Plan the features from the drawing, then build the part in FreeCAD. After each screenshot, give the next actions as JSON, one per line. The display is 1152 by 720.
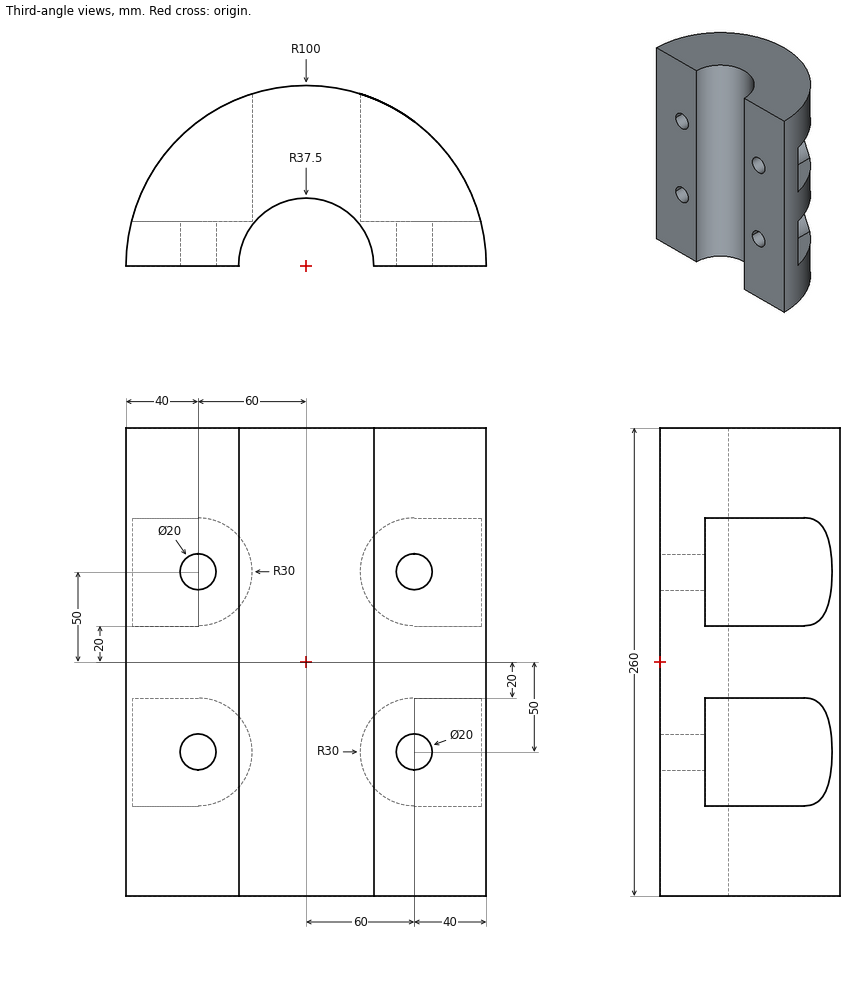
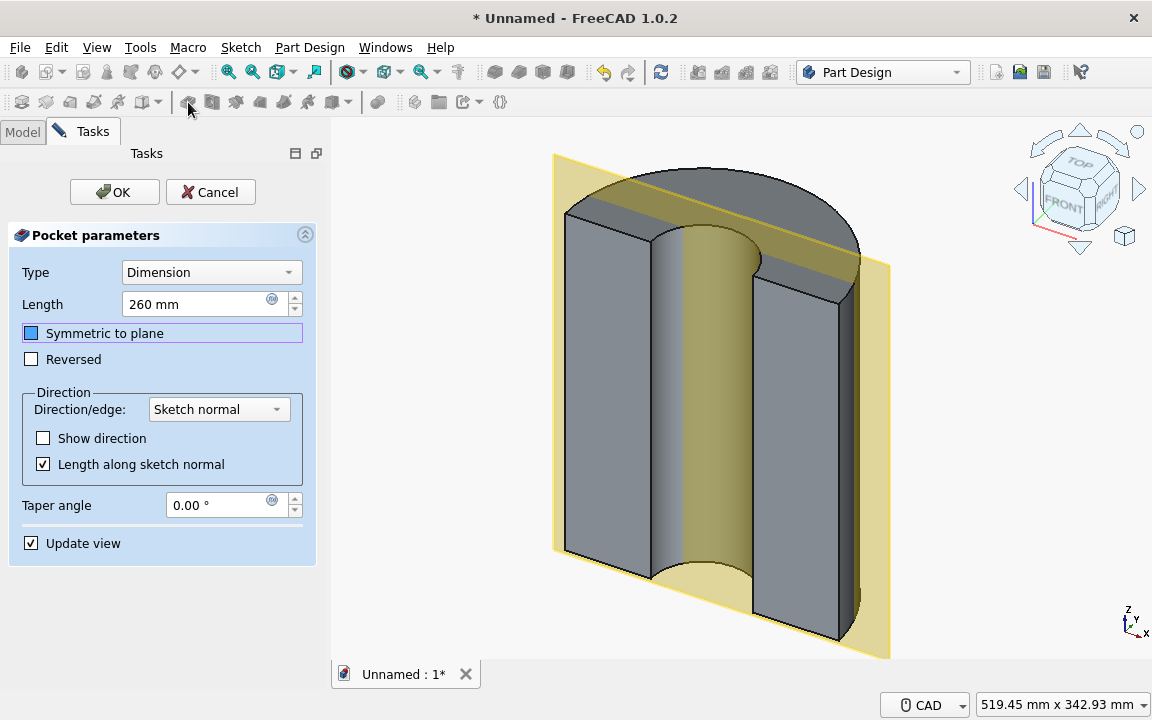
{"action": "left_click", "coordinate": [115, 192]}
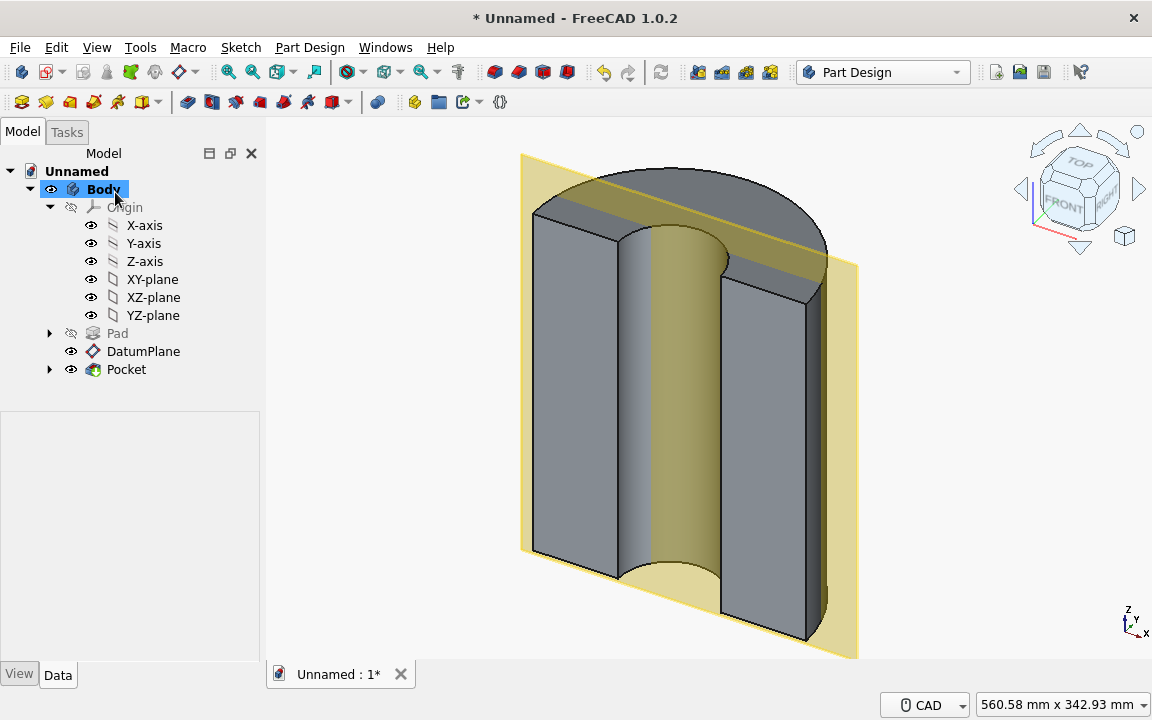
{"action": "left_click", "coordinate": [116, 351]}
{"action": "key", "text": "space"}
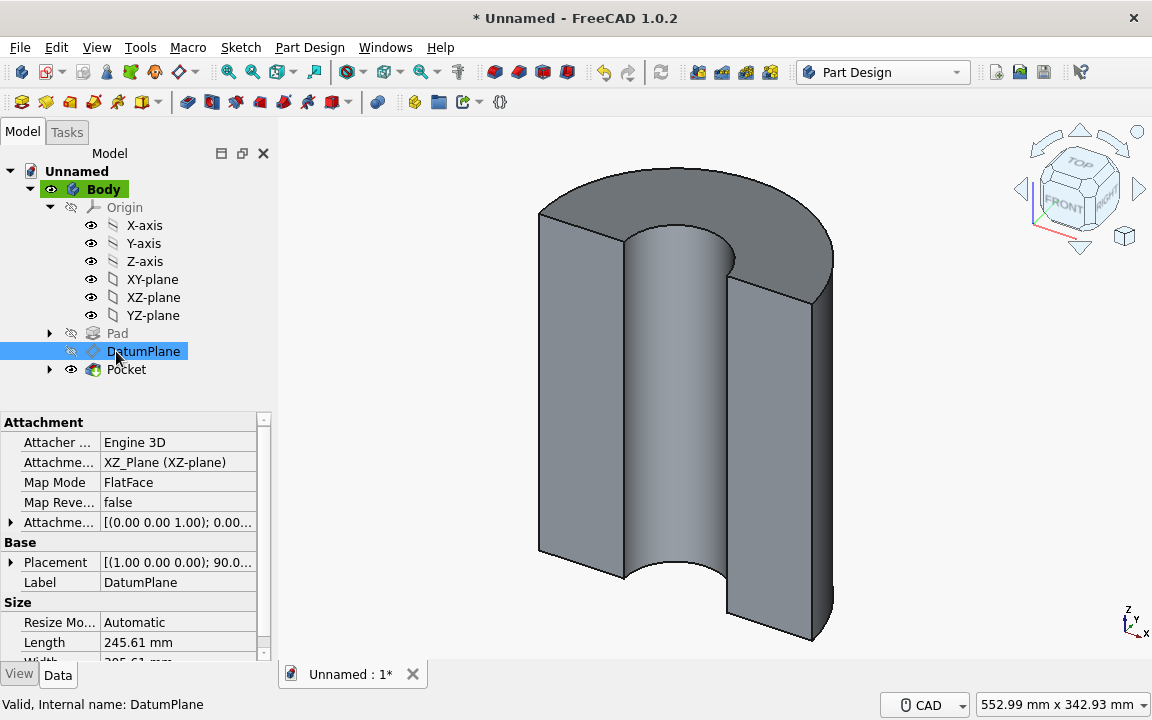
{"action": "left_click", "coordinate": [116, 369]}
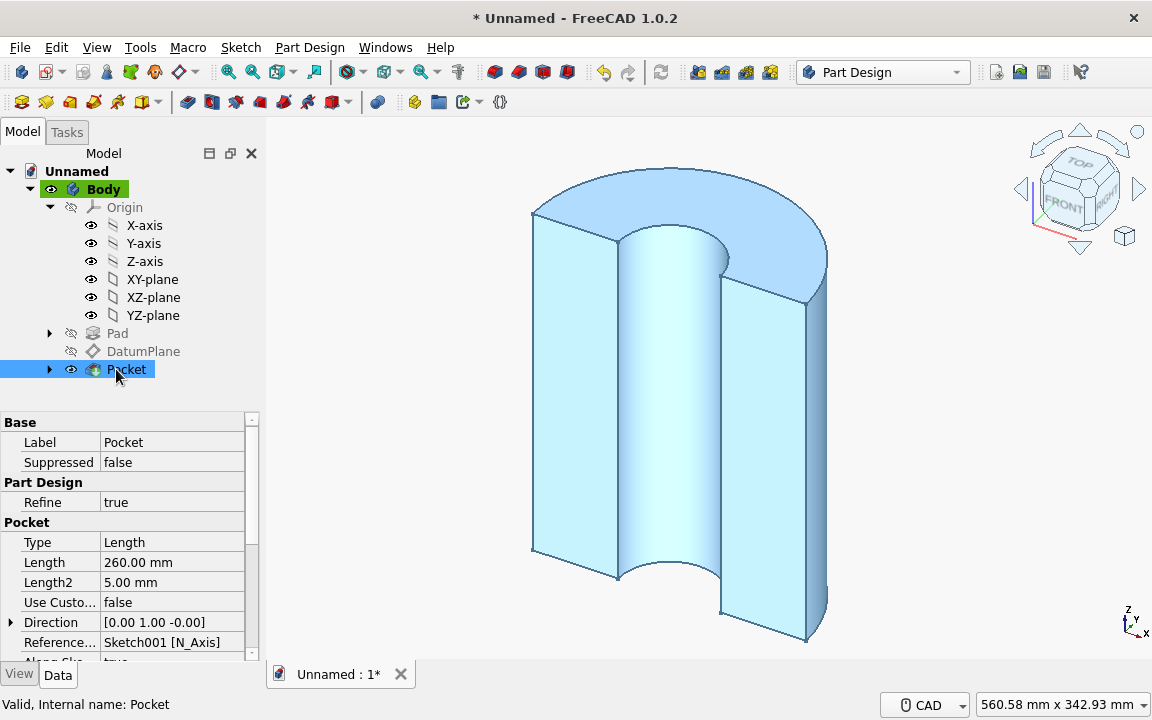
{"action": "left_click", "coordinate": [698, 72]}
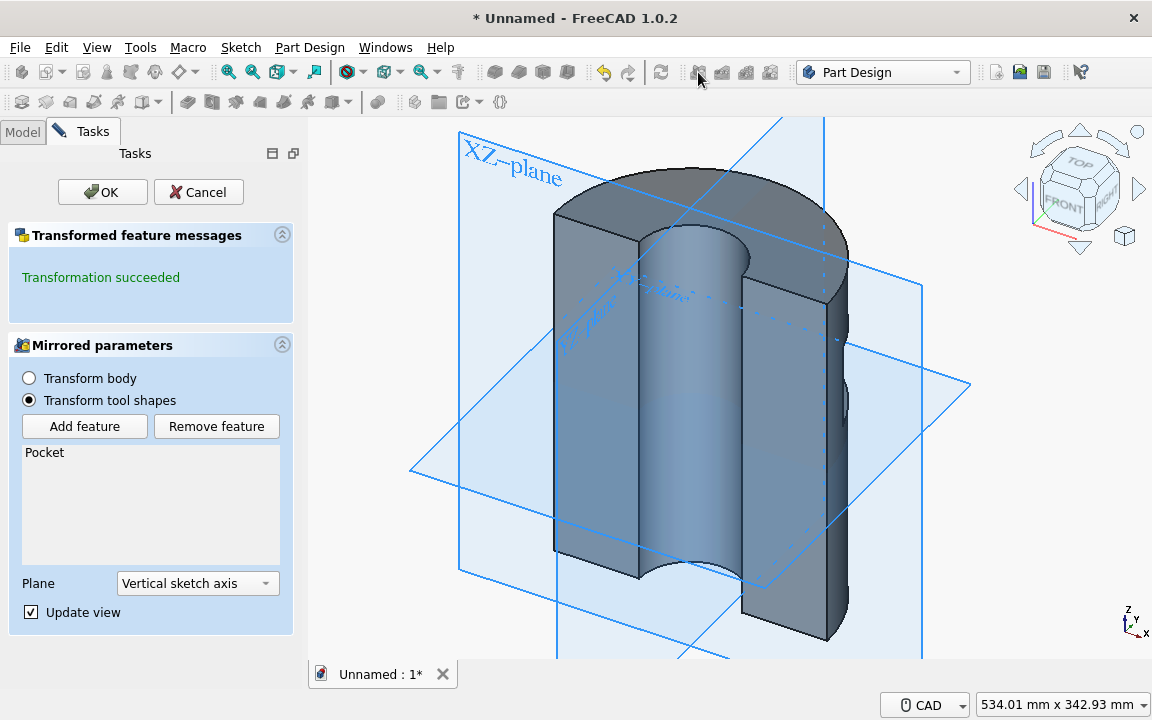
{"action": "left_click", "coordinate": [198, 584]}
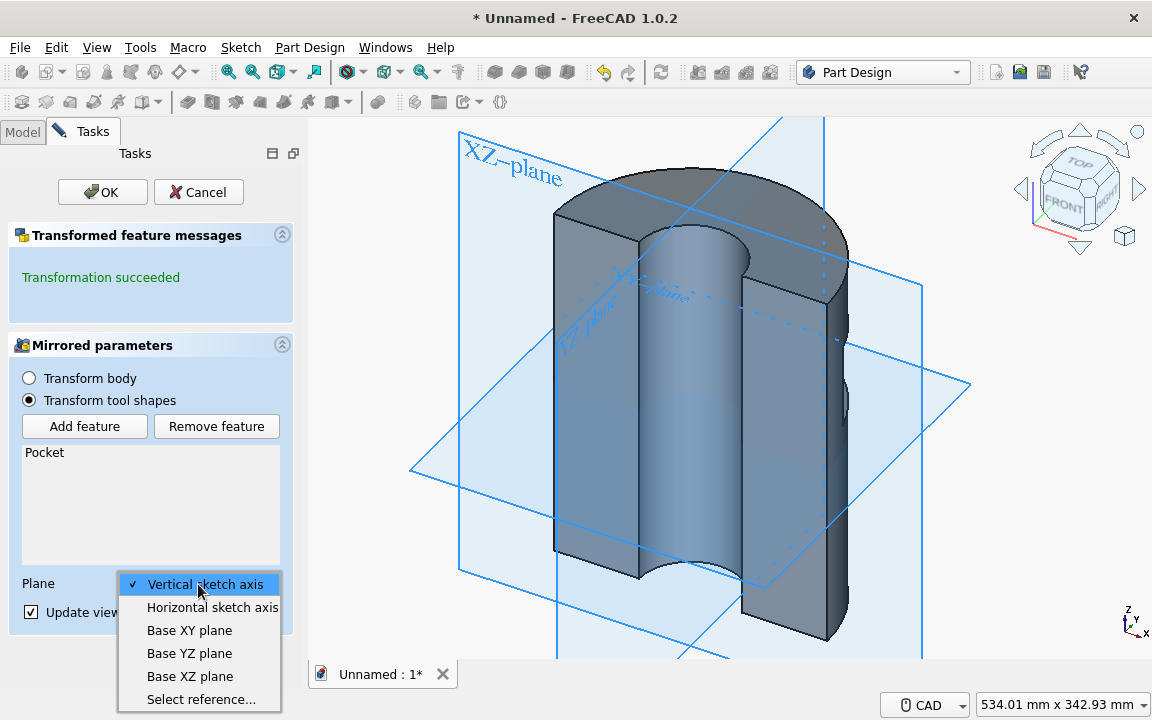
{"action": "left_click", "coordinate": [198, 630]}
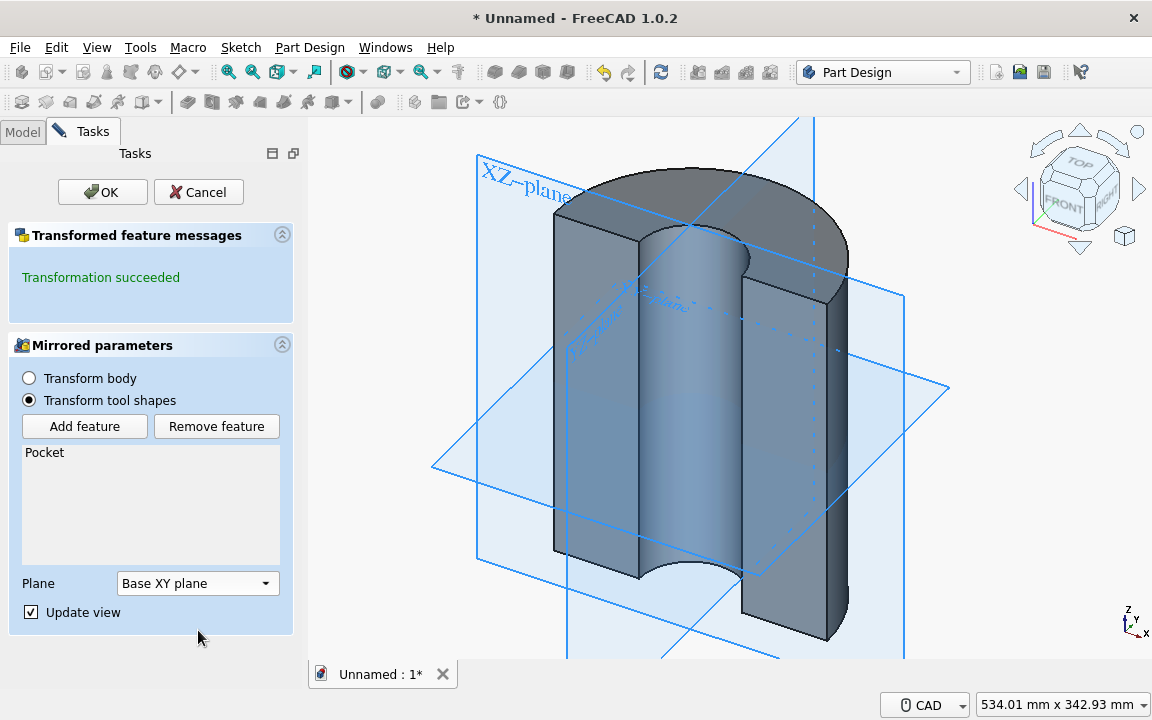
{"action": "left_click", "coordinate": [103, 192]}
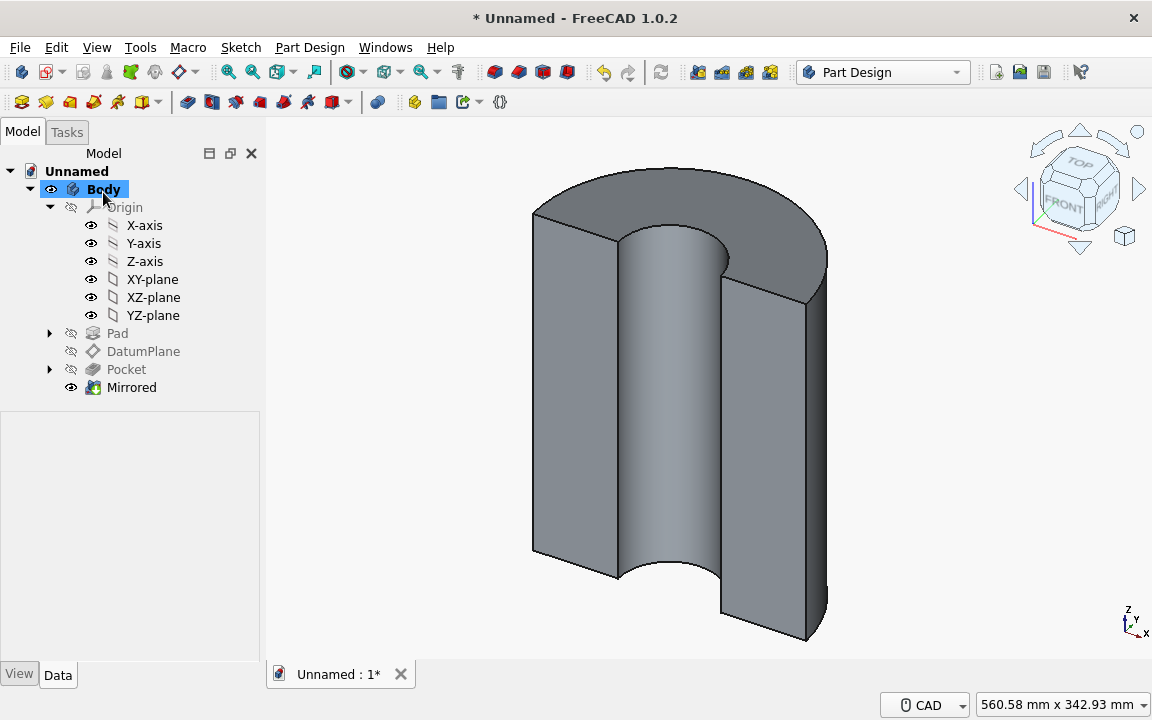
{"action": "left_click", "coordinate": [116, 369]}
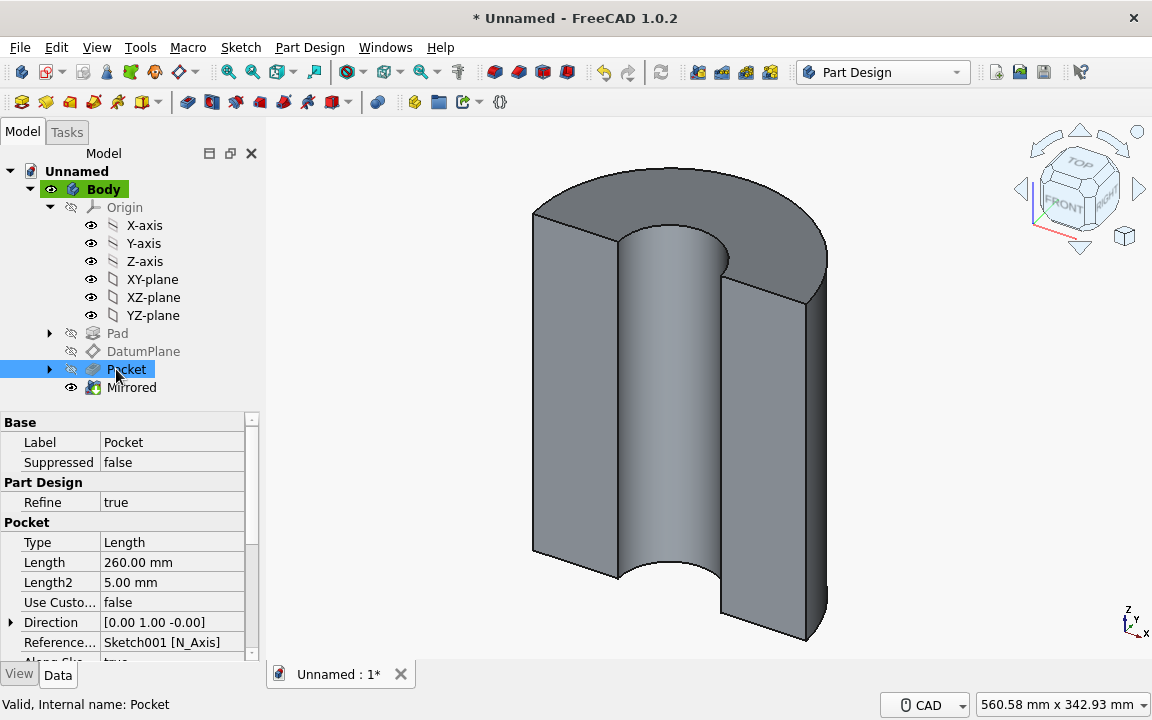
{"action": "left_click", "coordinate": [698, 72]}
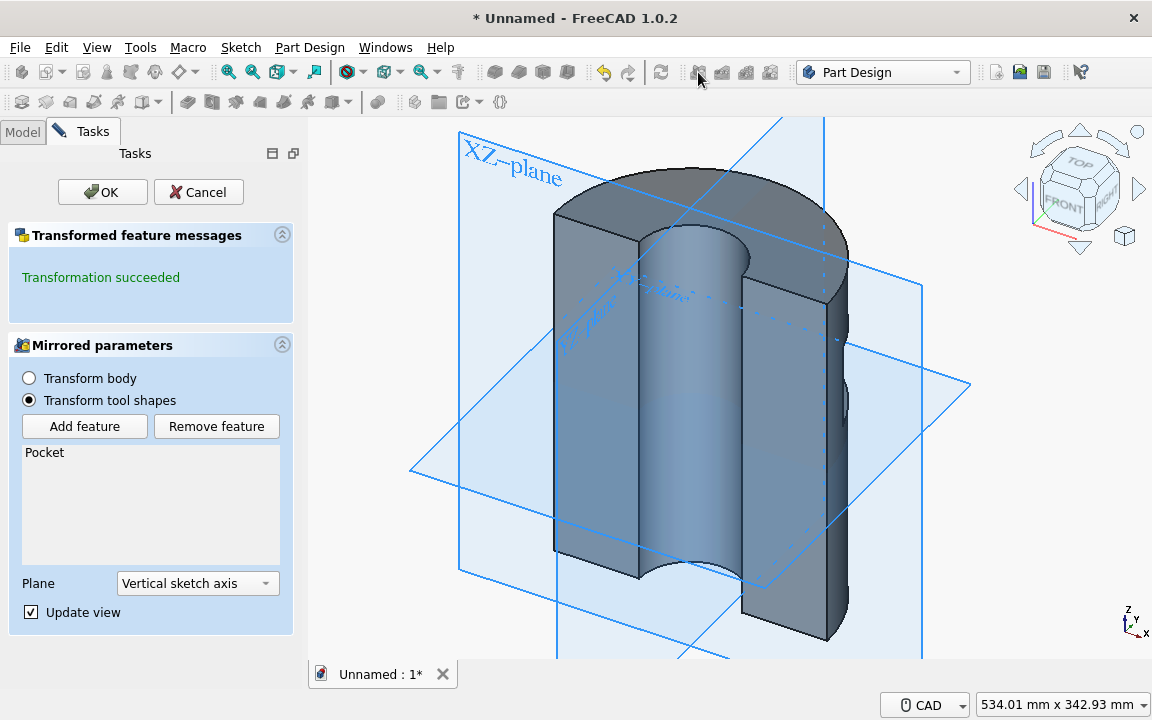
{"action": "left_click", "coordinate": [198, 584]}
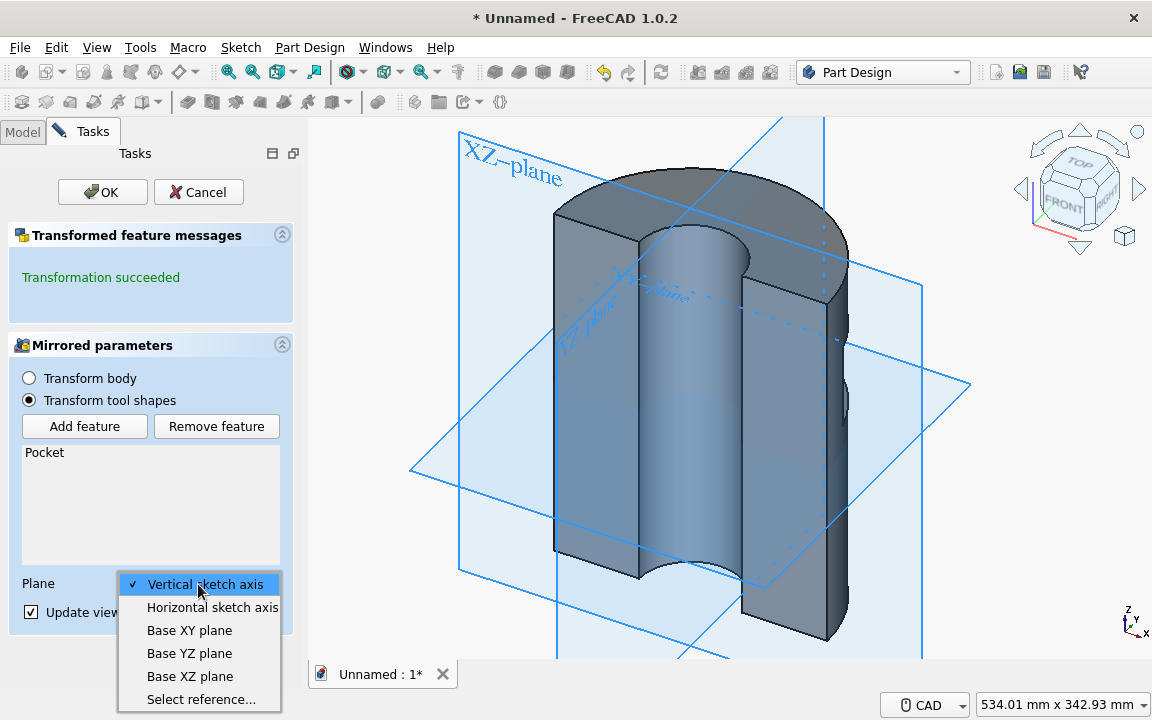
{"action": "left_click", "coordinate": [198, 654]}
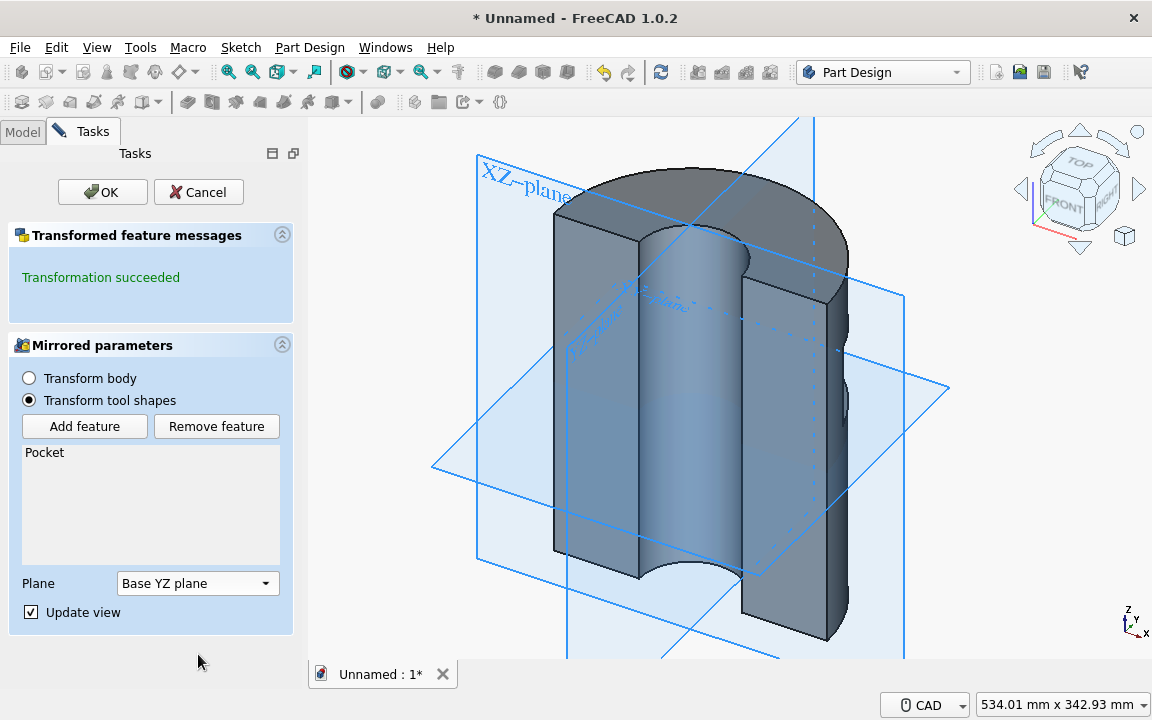
{"action": "left_click", "coordinate": [103, 192]}